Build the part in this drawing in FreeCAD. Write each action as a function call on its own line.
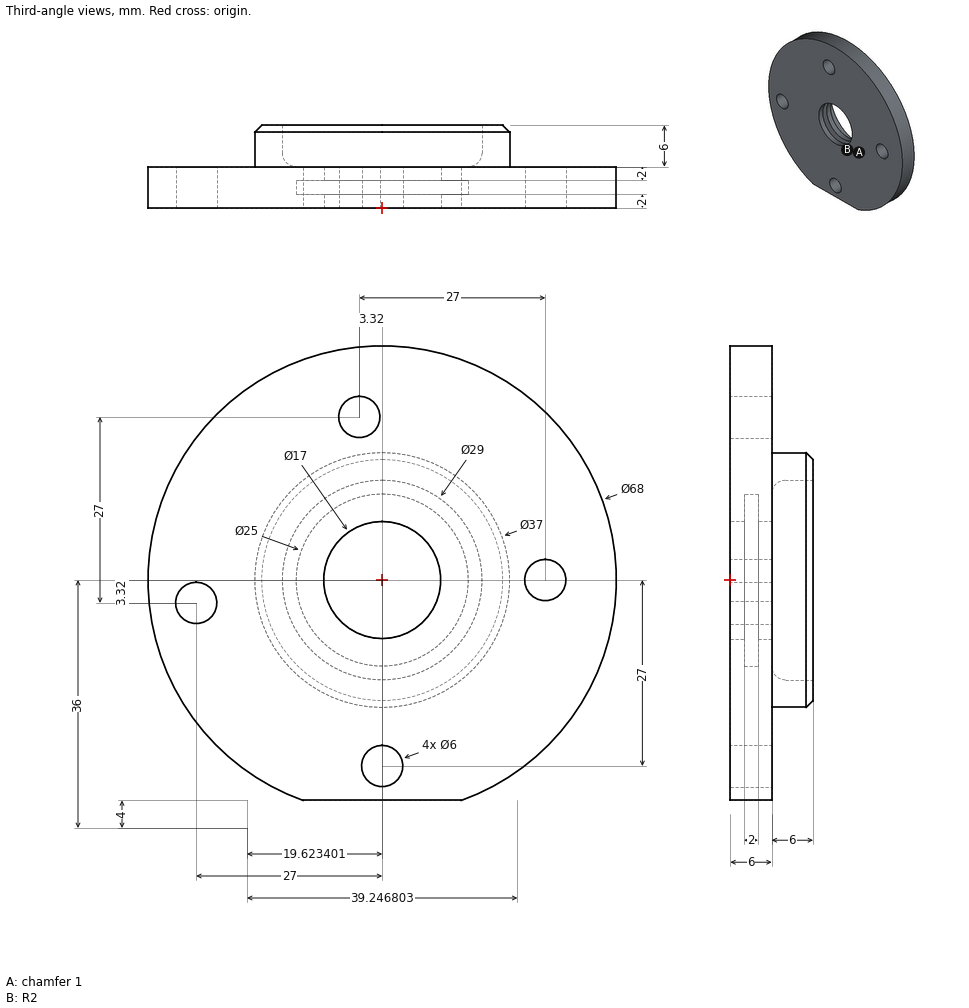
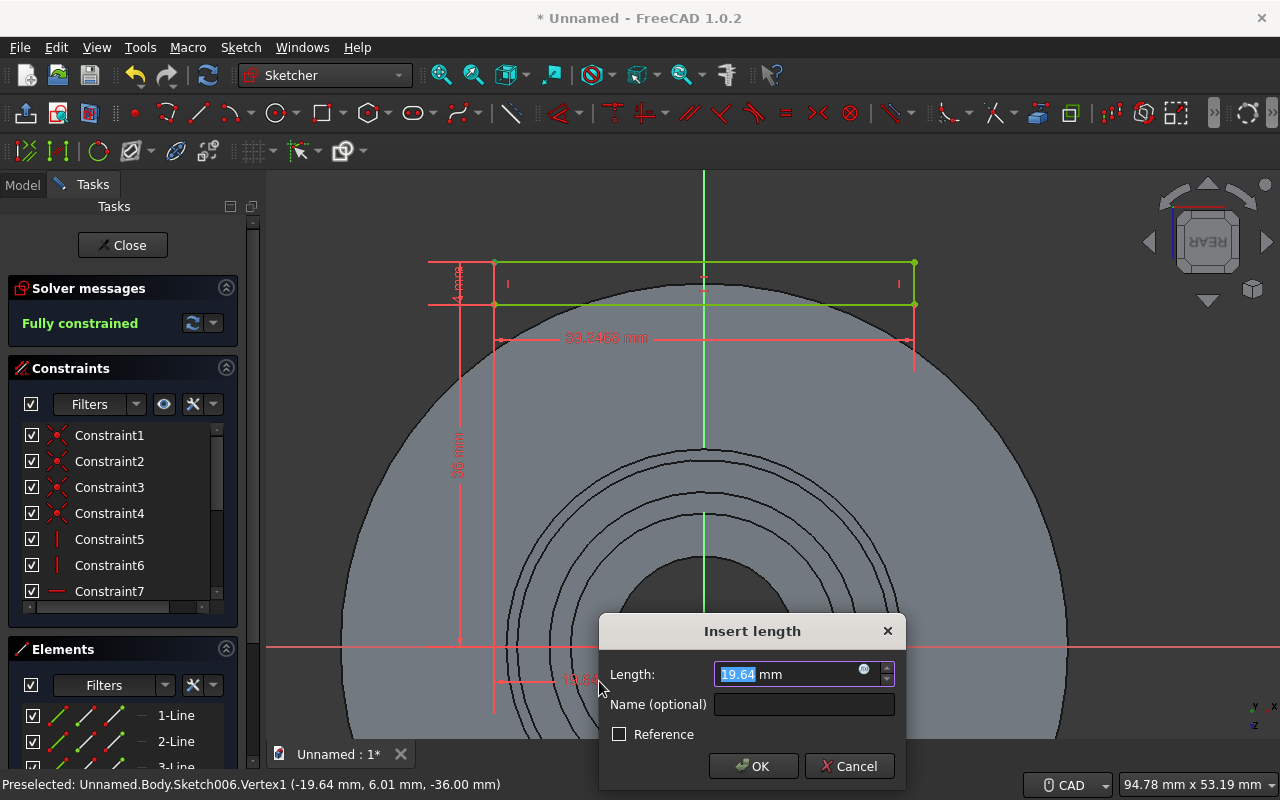
text(19.623401)
key(Return)
key(Escape)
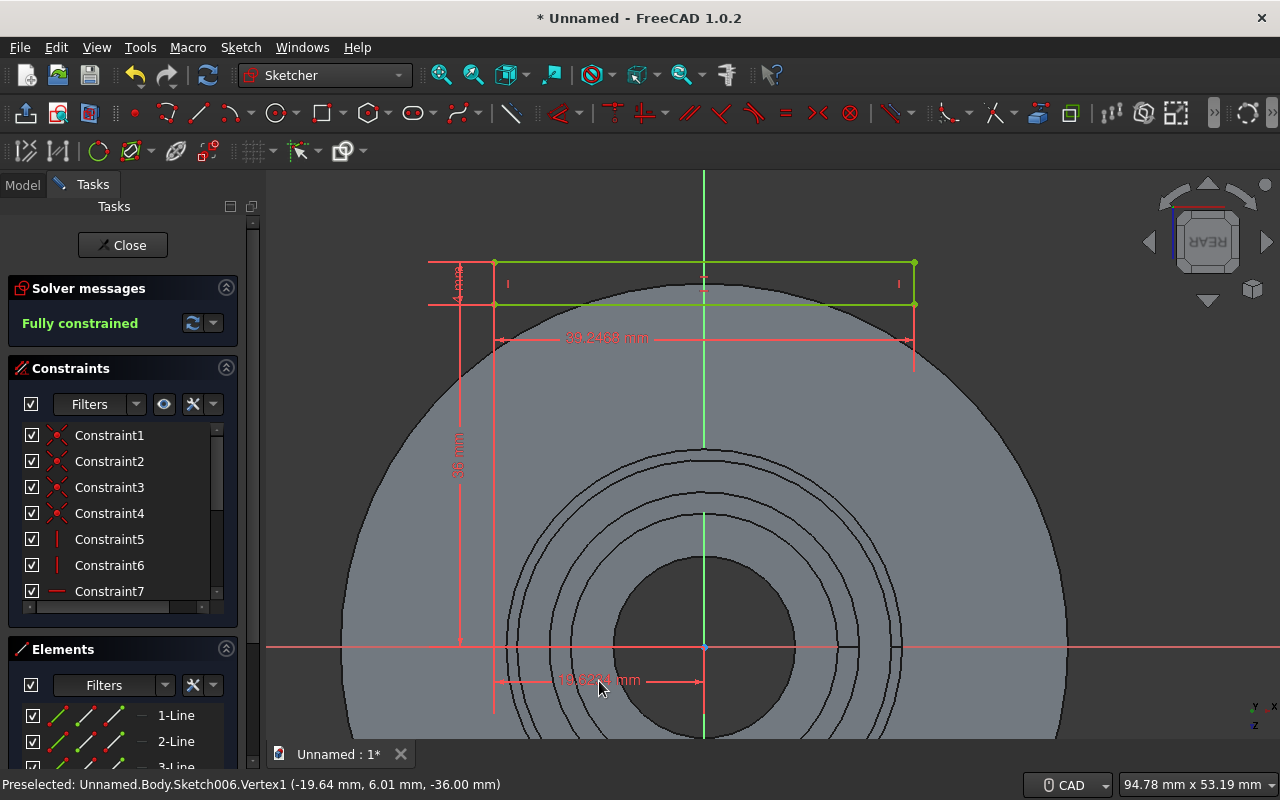
click(123, 245)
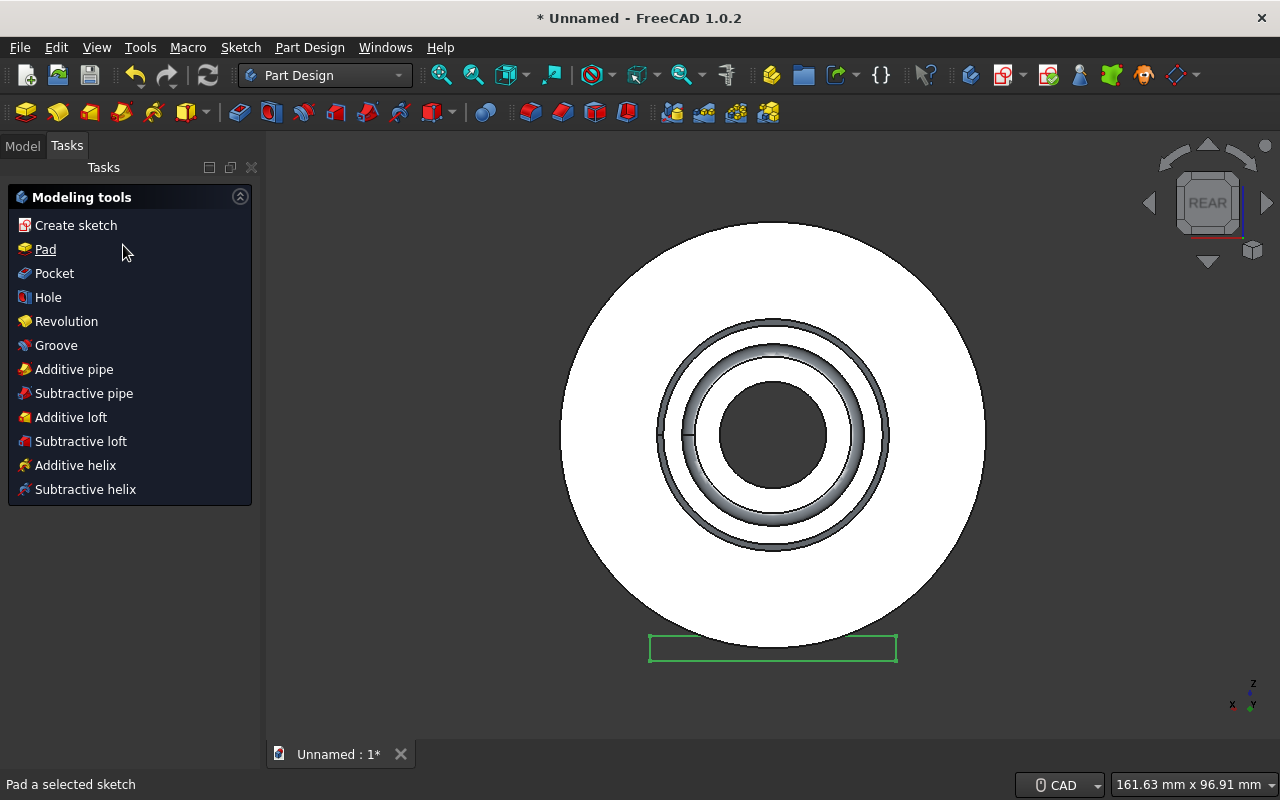
click(240, 112)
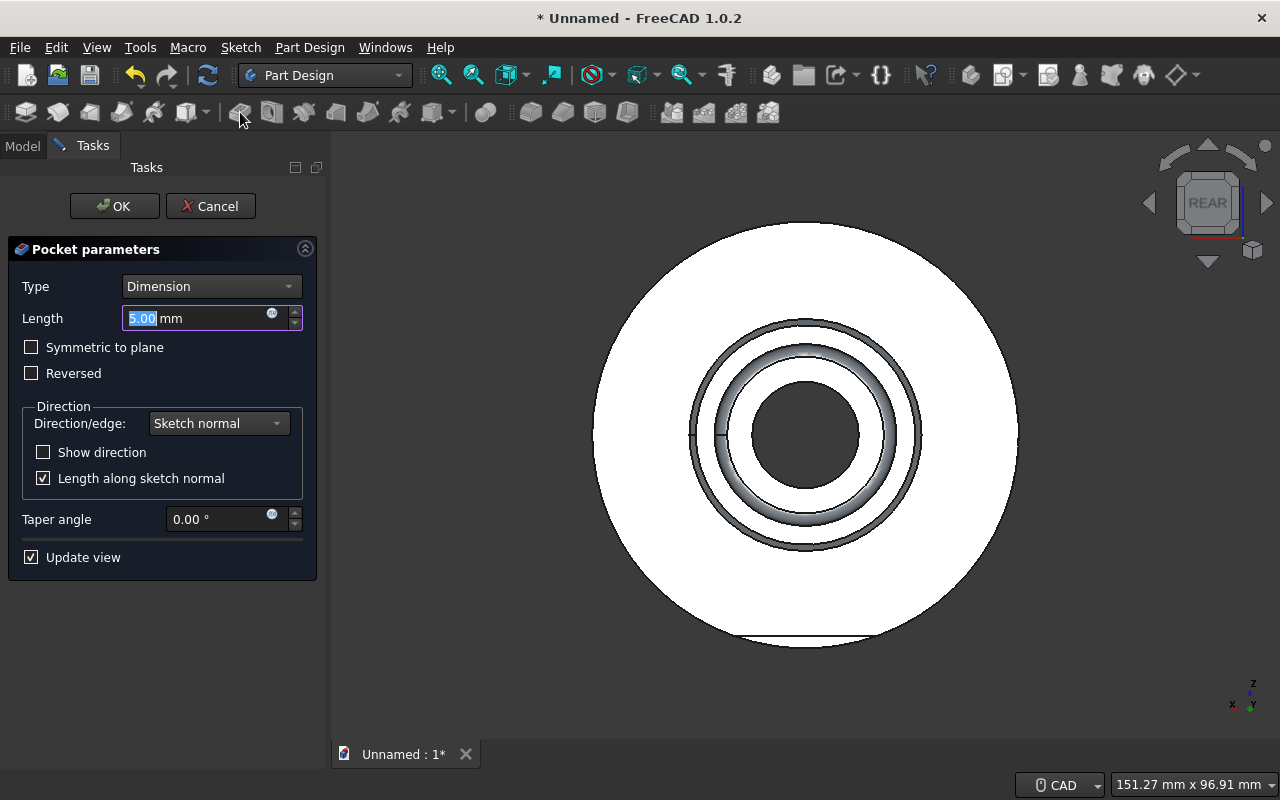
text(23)
key(Tab)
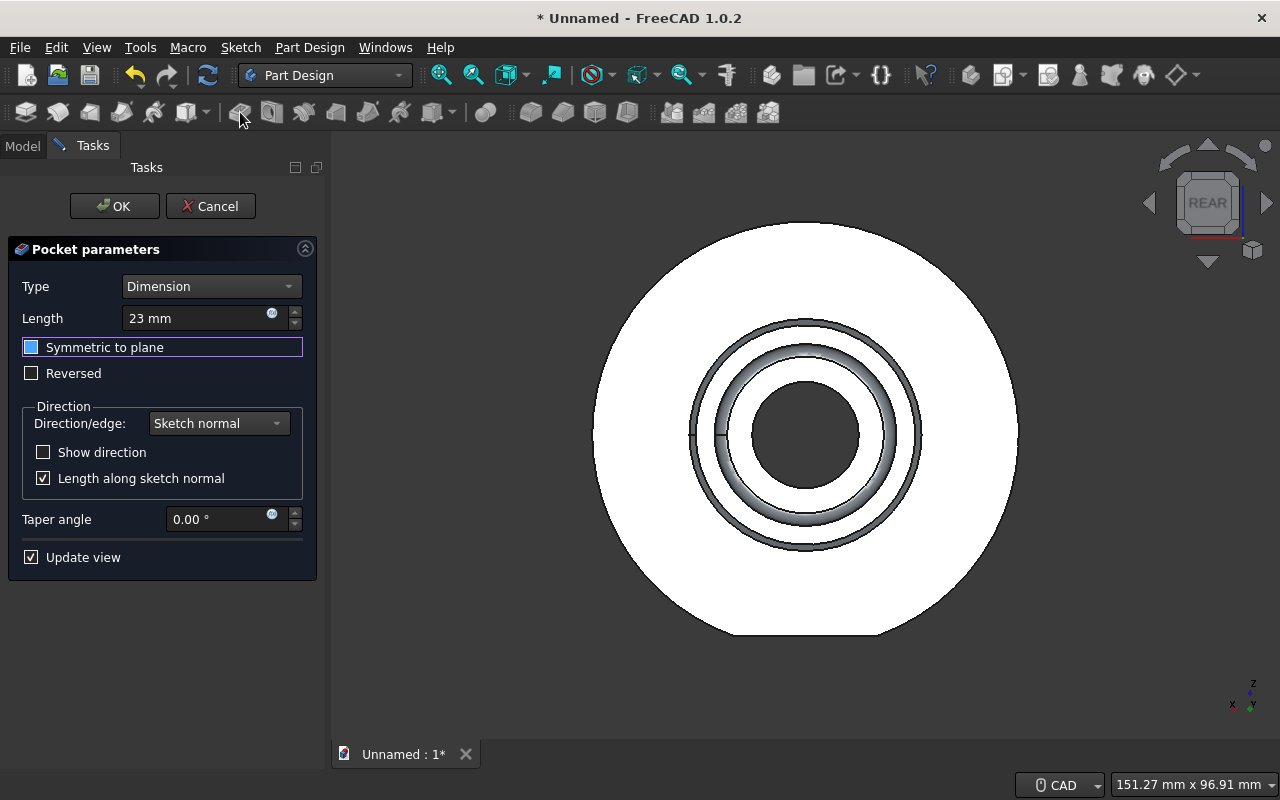
click(115, 206)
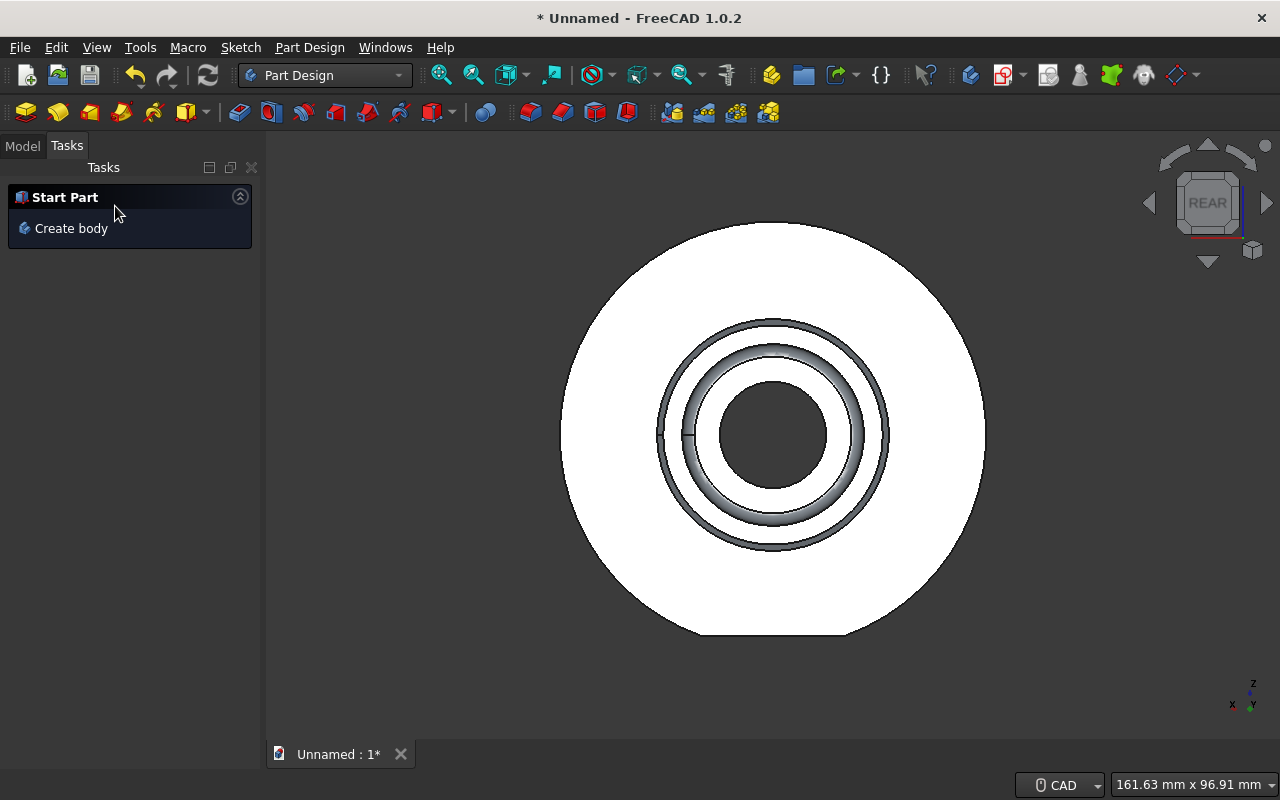
click(651, 546)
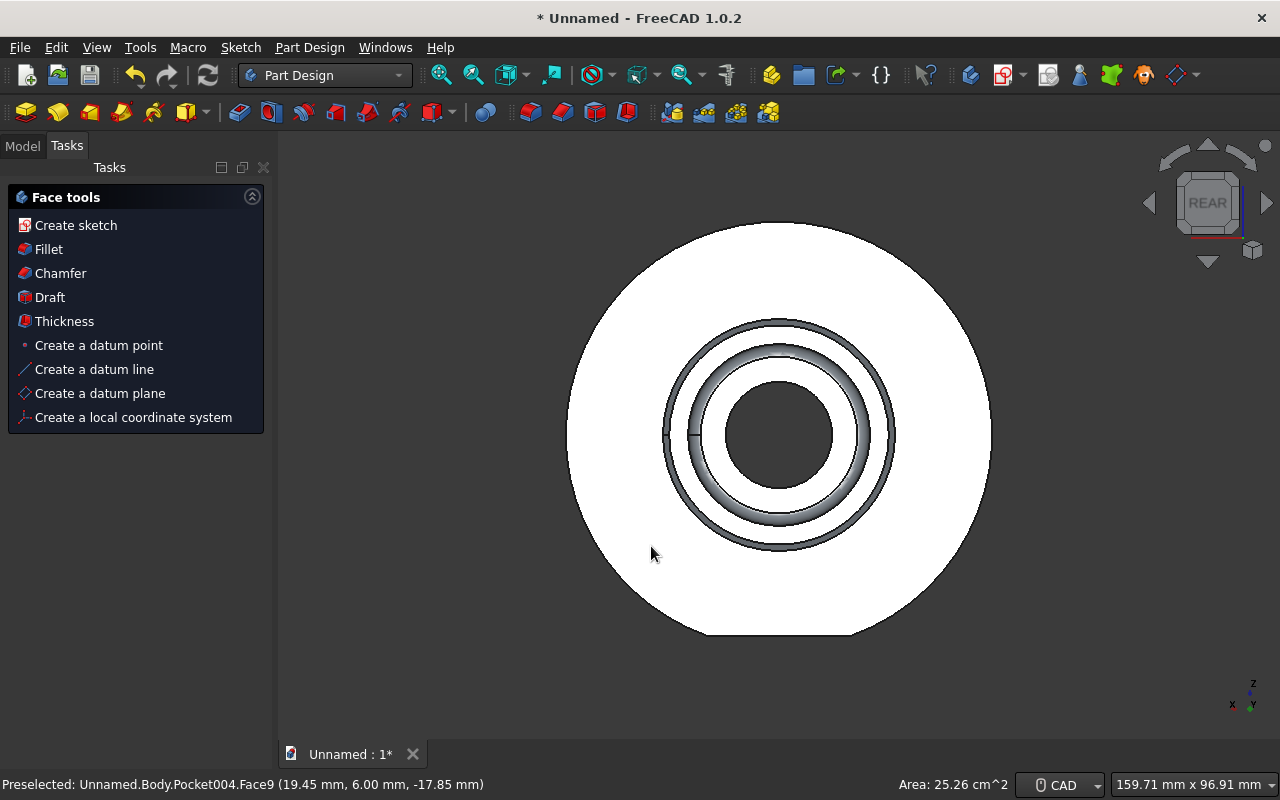
click(1004, 76)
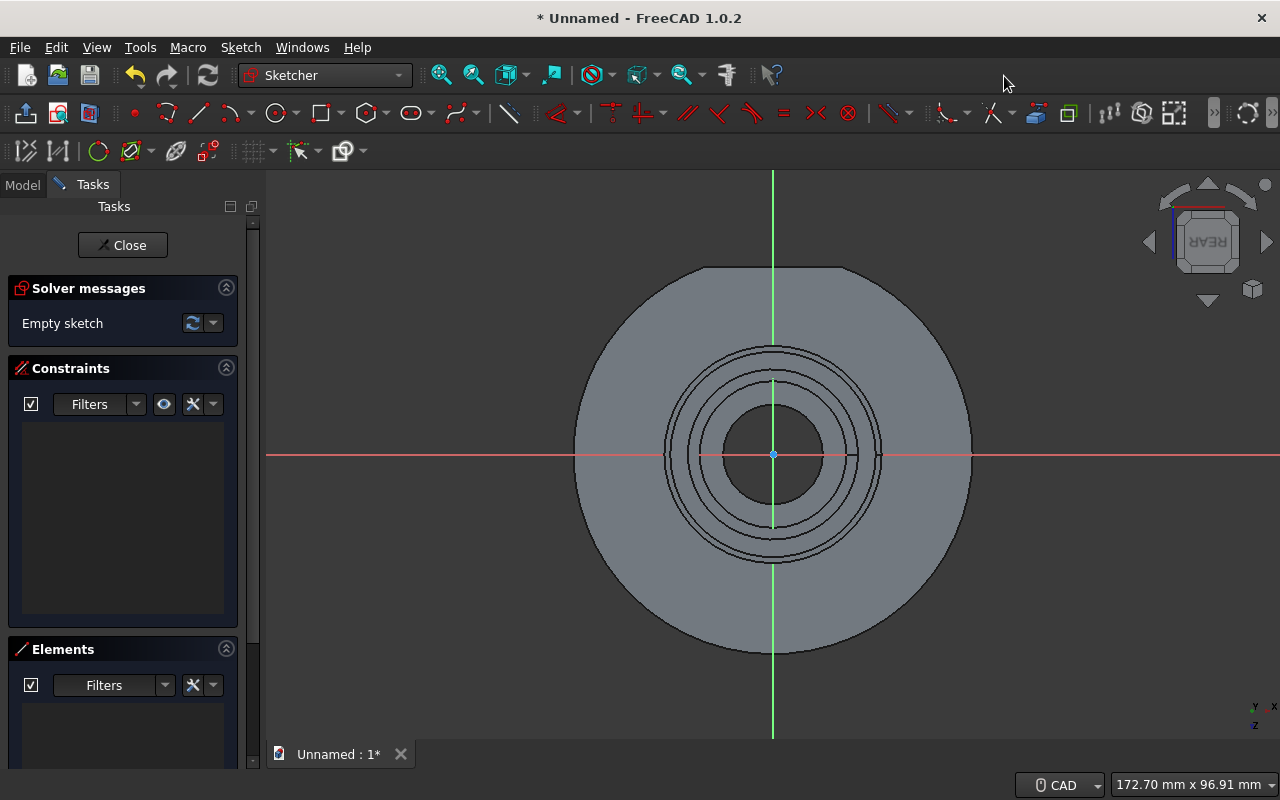
click(276, 114)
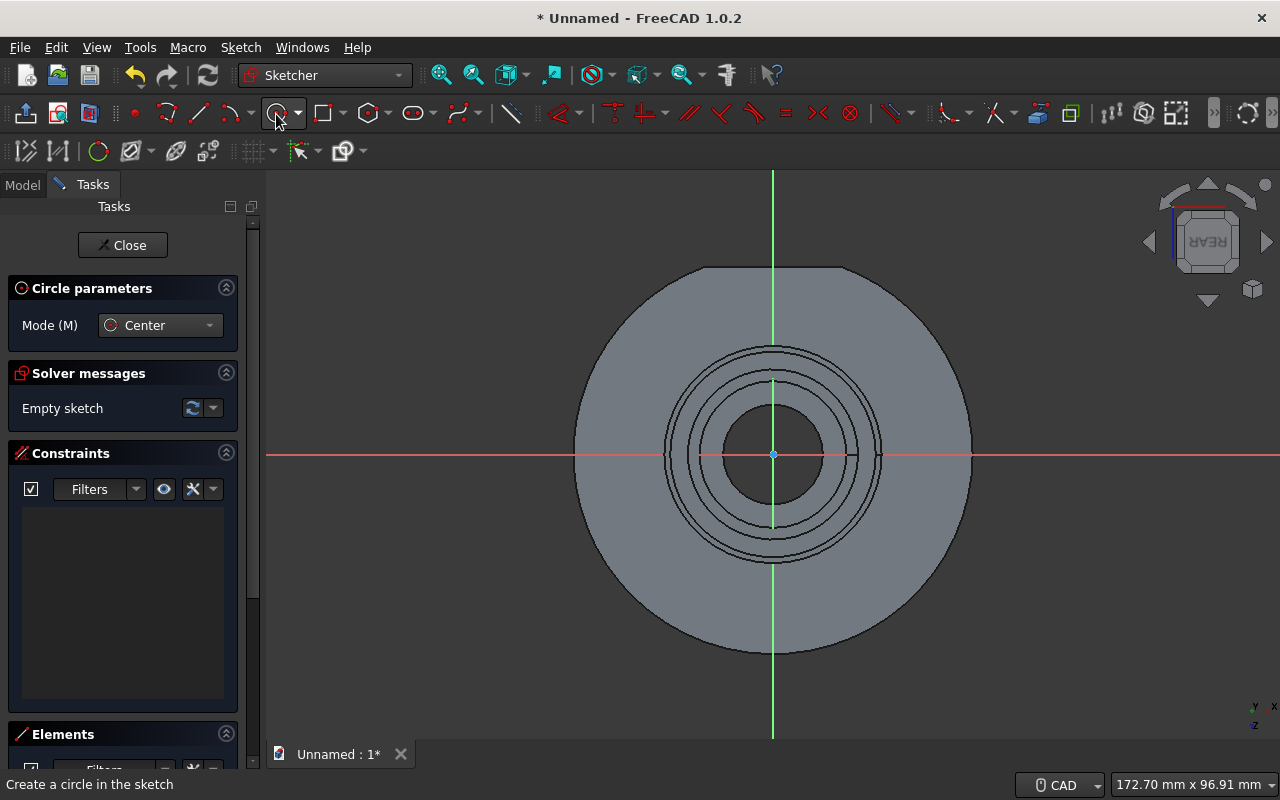
scroll(773, 296, up, 2)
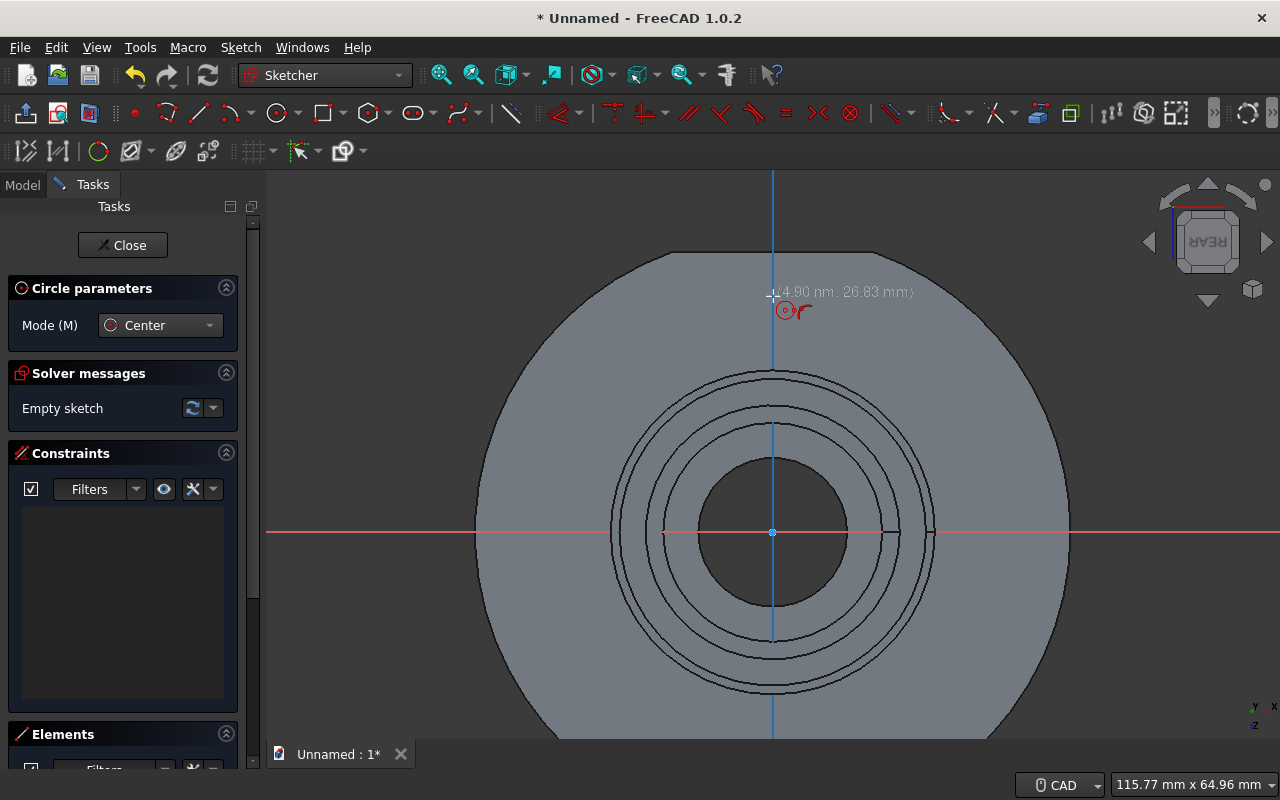
click(773, 296)
click(791, 277)